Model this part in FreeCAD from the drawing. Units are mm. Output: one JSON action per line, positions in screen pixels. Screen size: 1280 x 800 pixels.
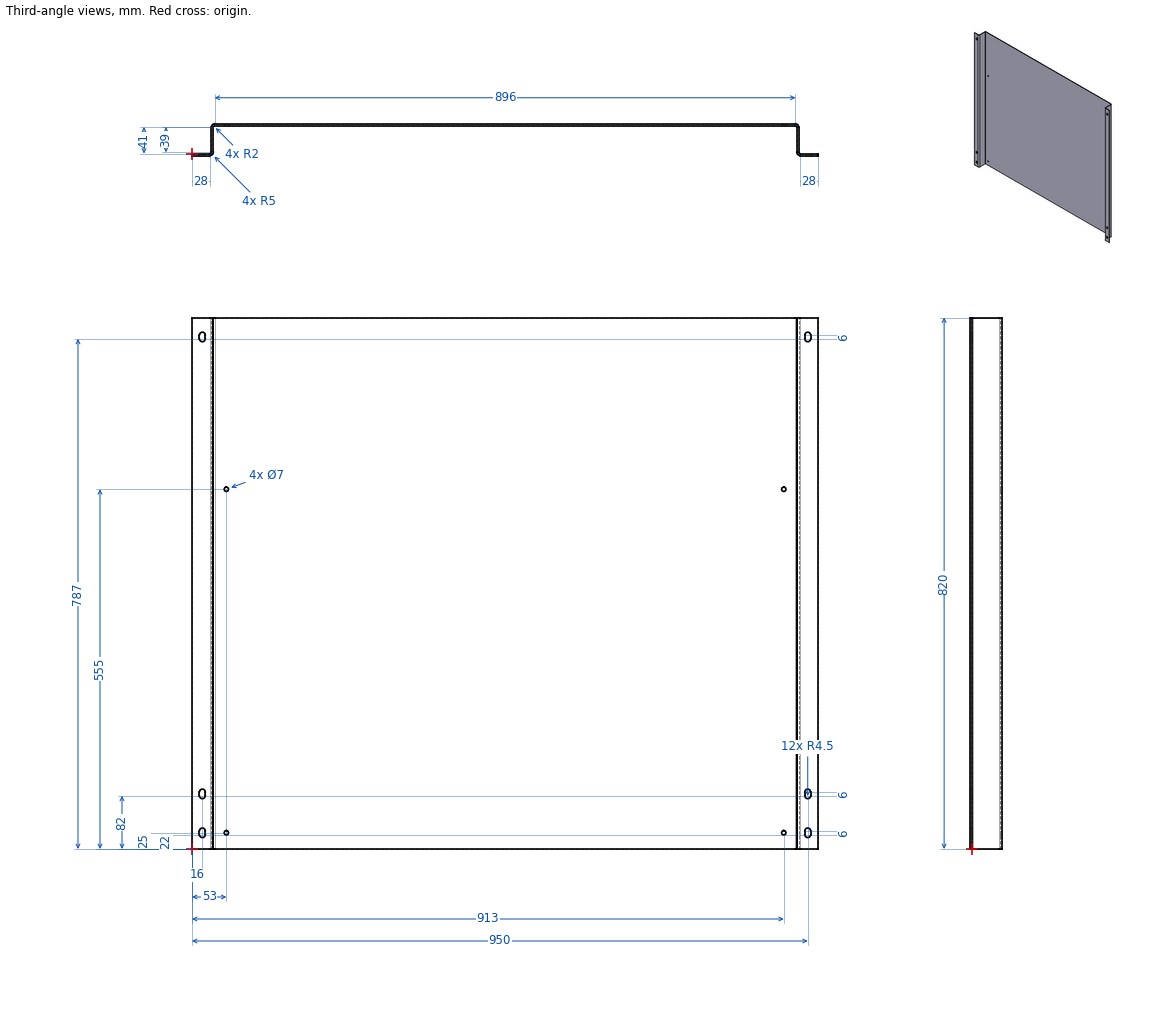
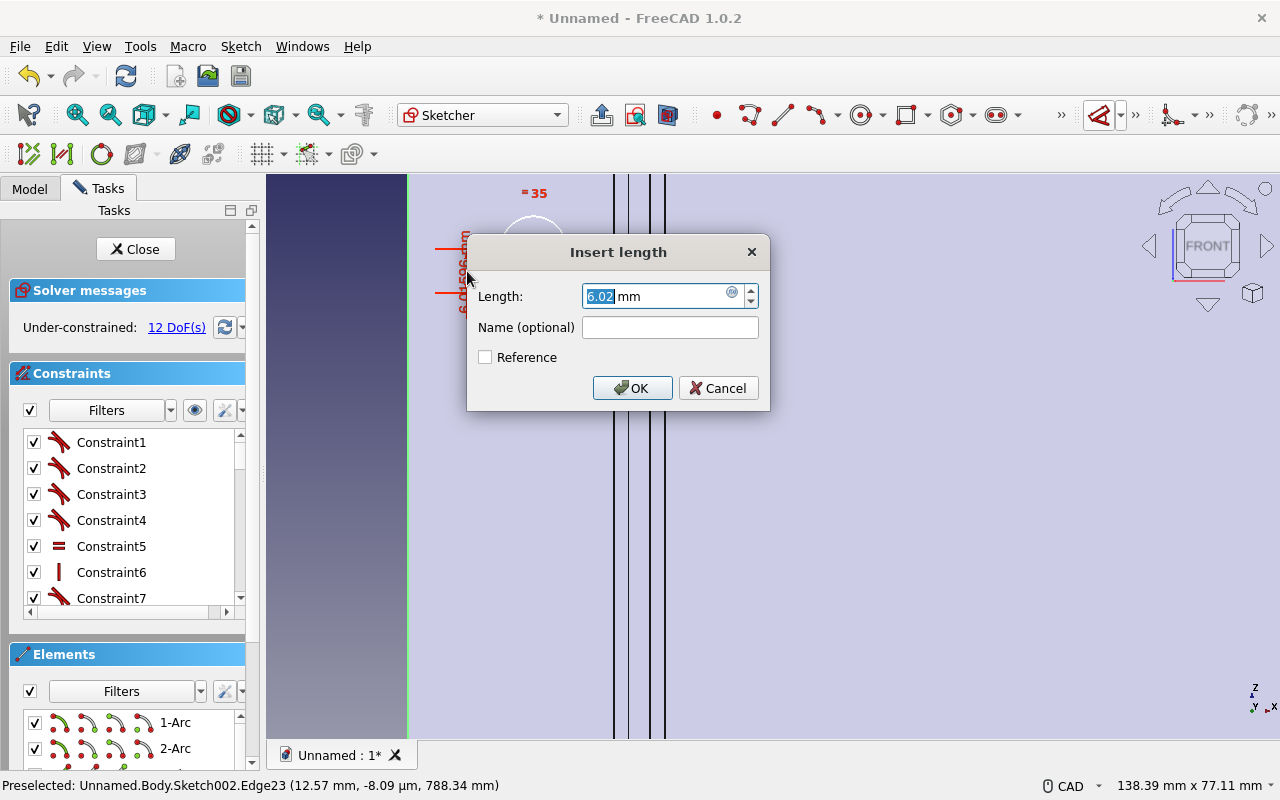
{"action": "type", "text": "6"}
{"action": "key", "text": "Return"}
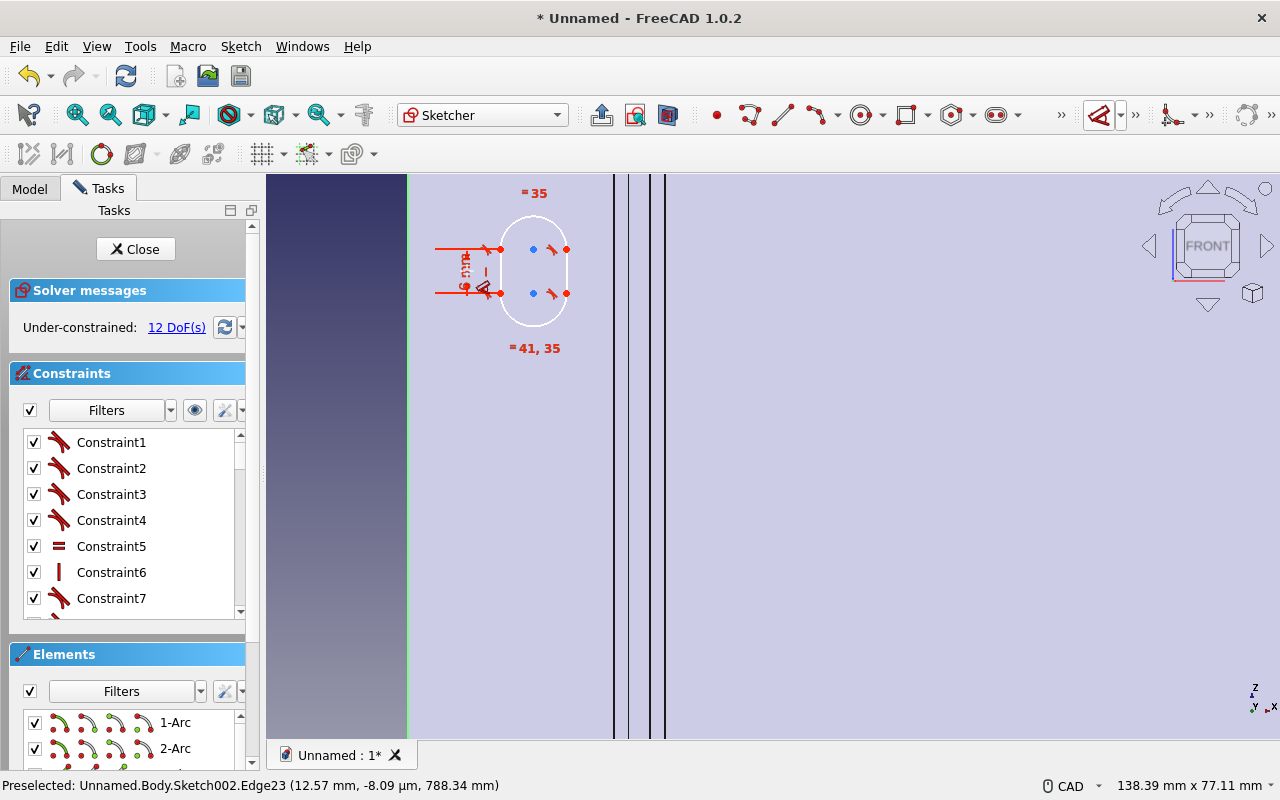
{"action": "scroll", "coordinate": [497, 283], "scroll_direction": "down", "scroll_amount": 14}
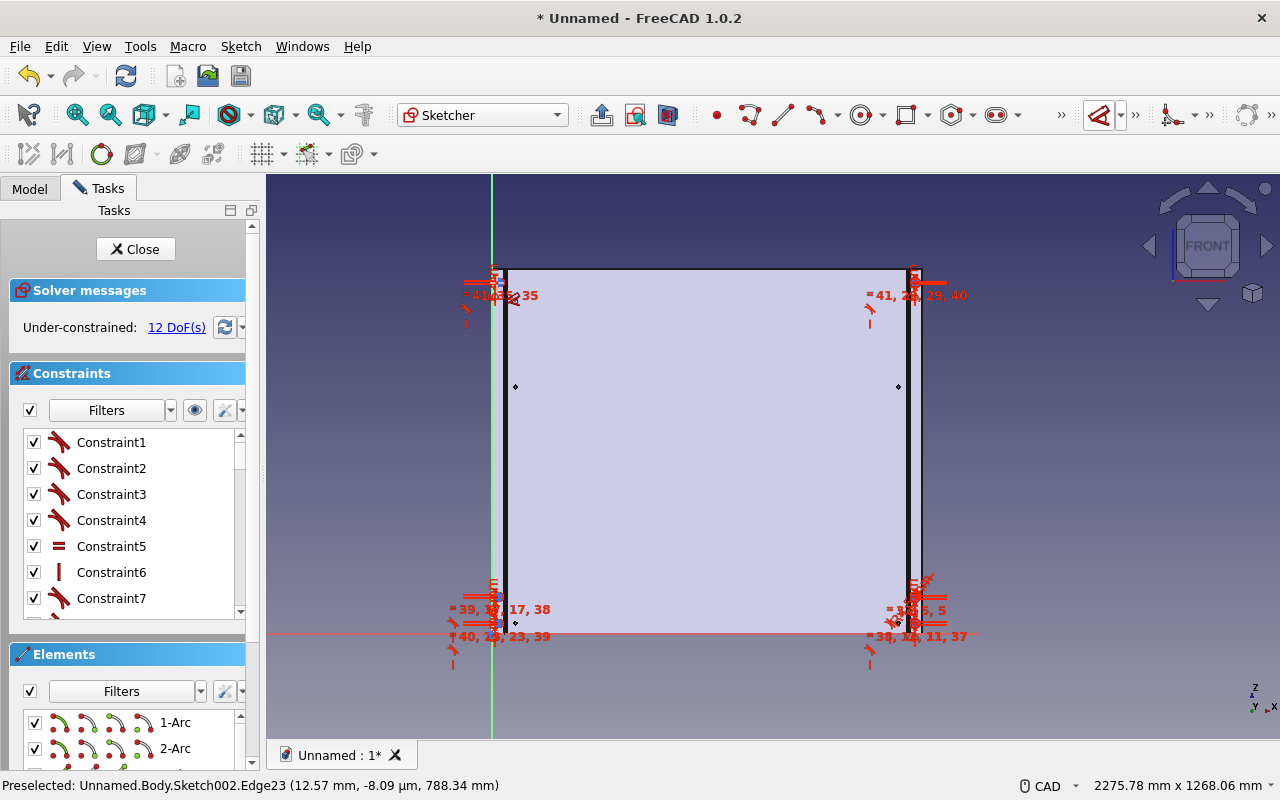
{"action": "scroll", "coordinate": [913, 599], "scroll_direction": "up", "scroll_amount": 10}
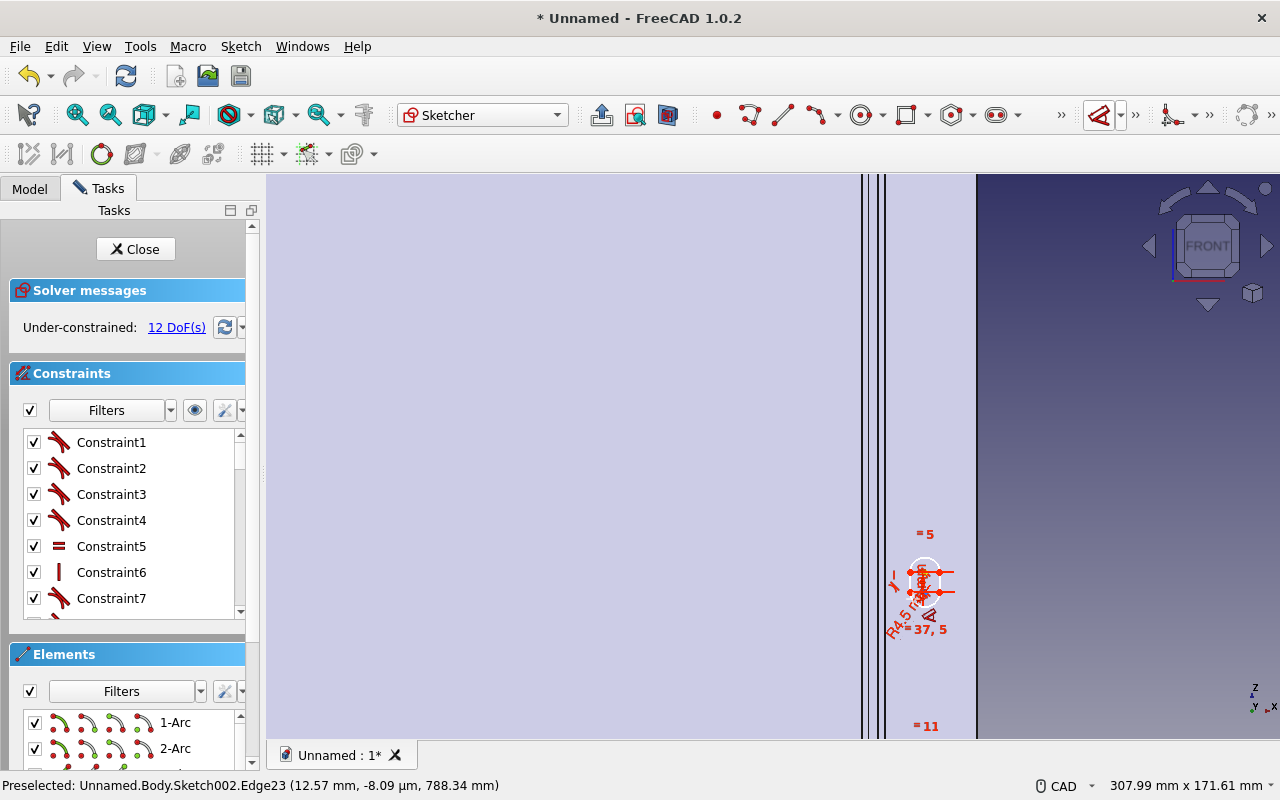
{"action": "left_click", "coordinate": [910, 592]}
{"action": "left_click", "coordinate": [944, 652]}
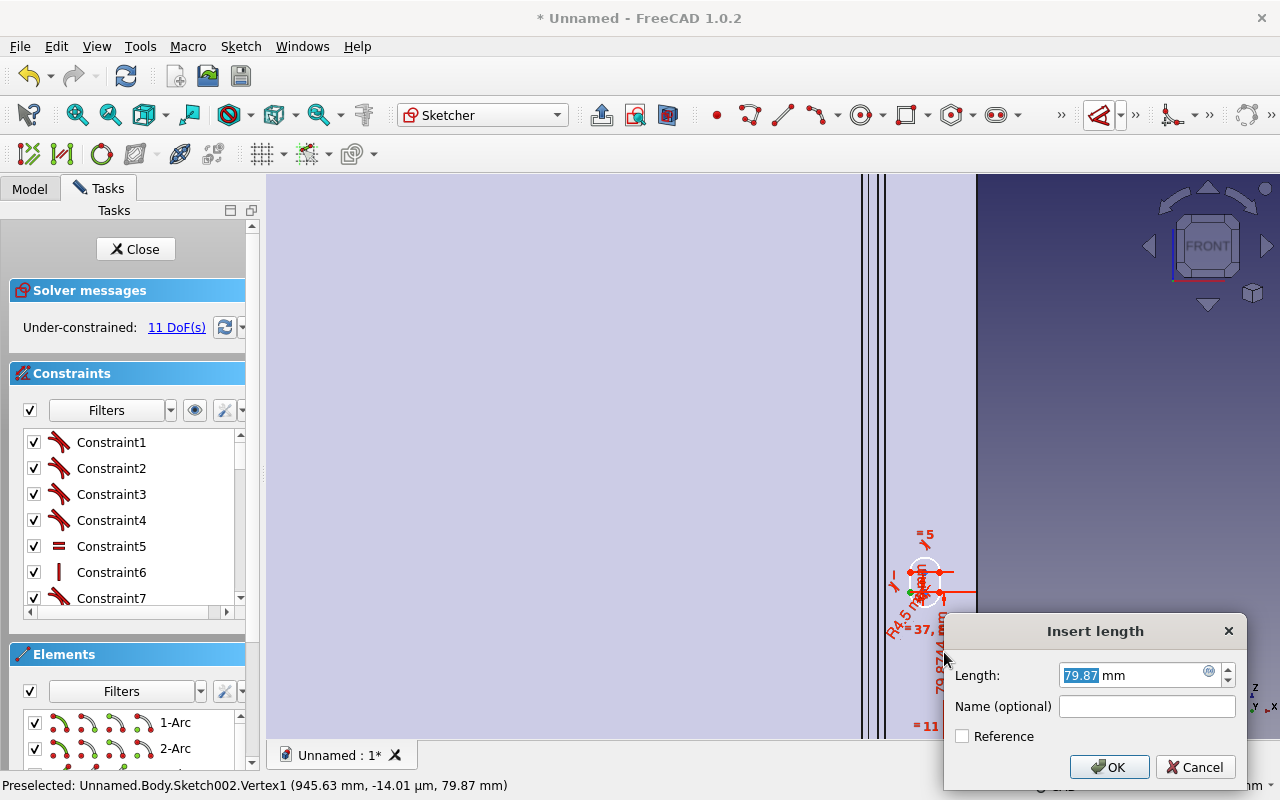
{"action": "type", "text": "82"}
{"action": "key", "text": "Return"}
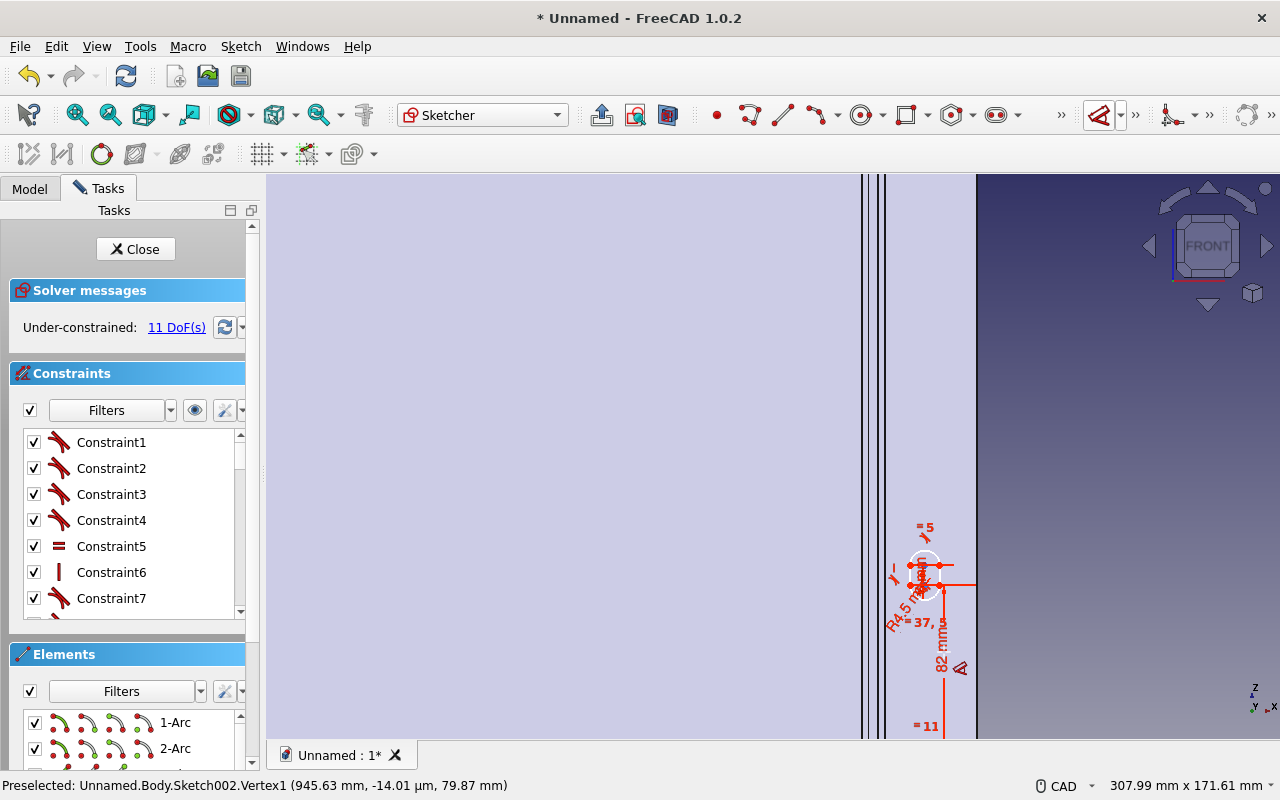
{"action": "scroll", "coordinate": [914, 600], "scroll_direction": "down", "scroll_amount": 10}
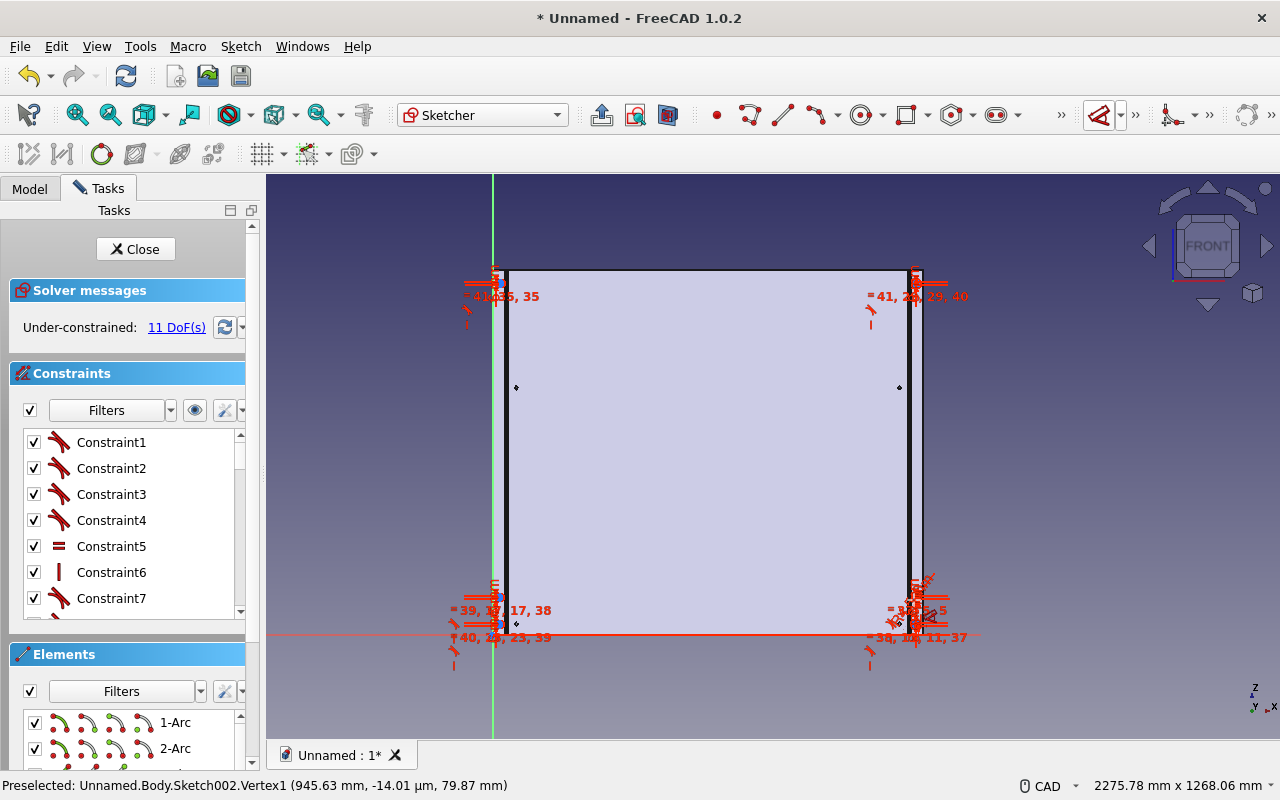
{"action": "scroll", "coordinate": [914, 626], "scroll_direction": "up", "scroll_amount": 10}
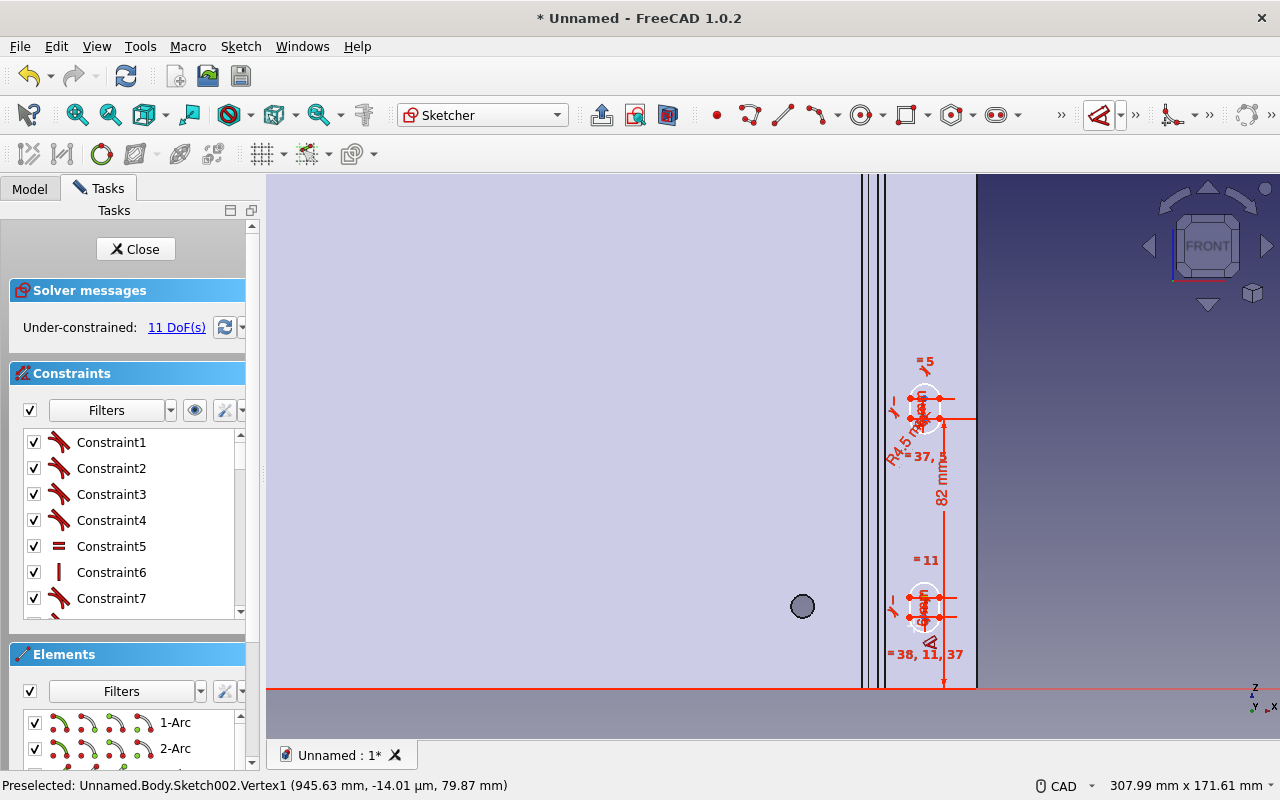
{"action": "left_click", "coordinate": [910, 617]}
{"action": "left_click", "coordinate": [944, 653]}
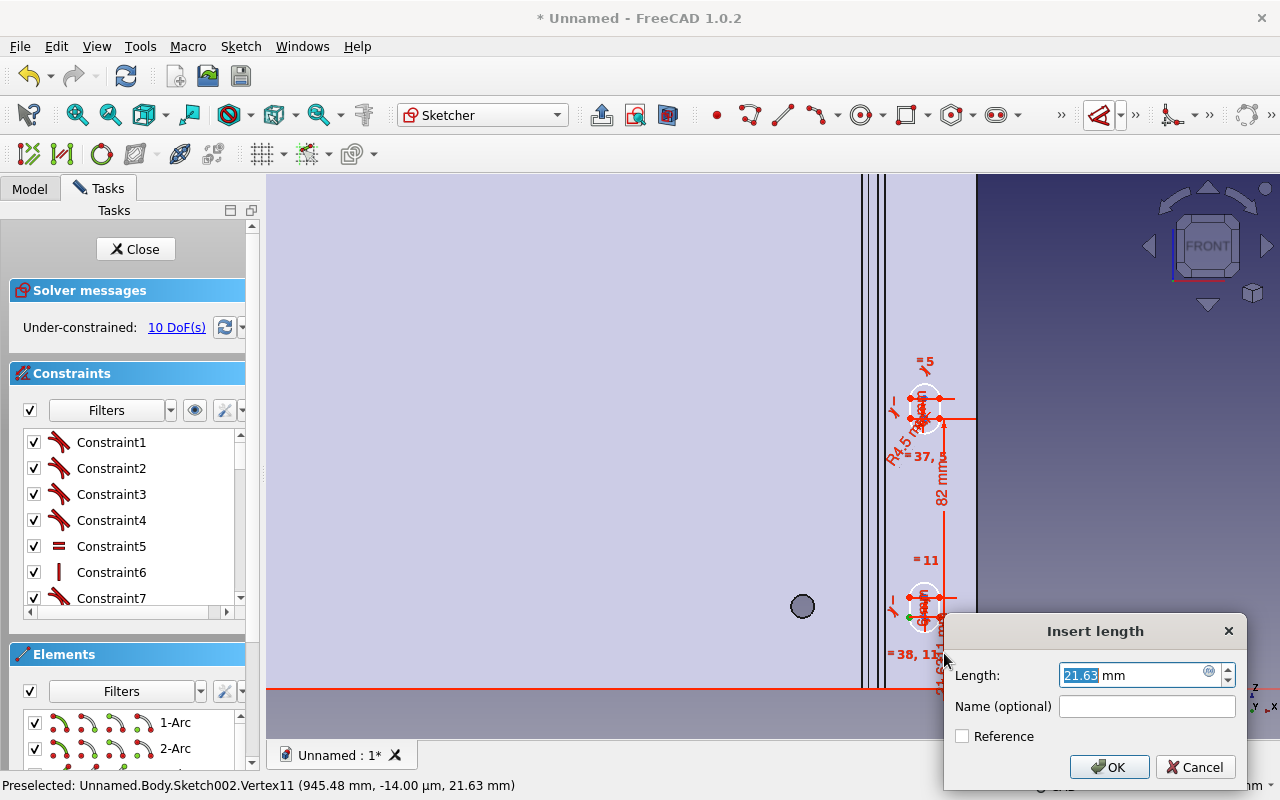
{"action": "type", "text": "22"}
{"action": "key", "text": "Return"}